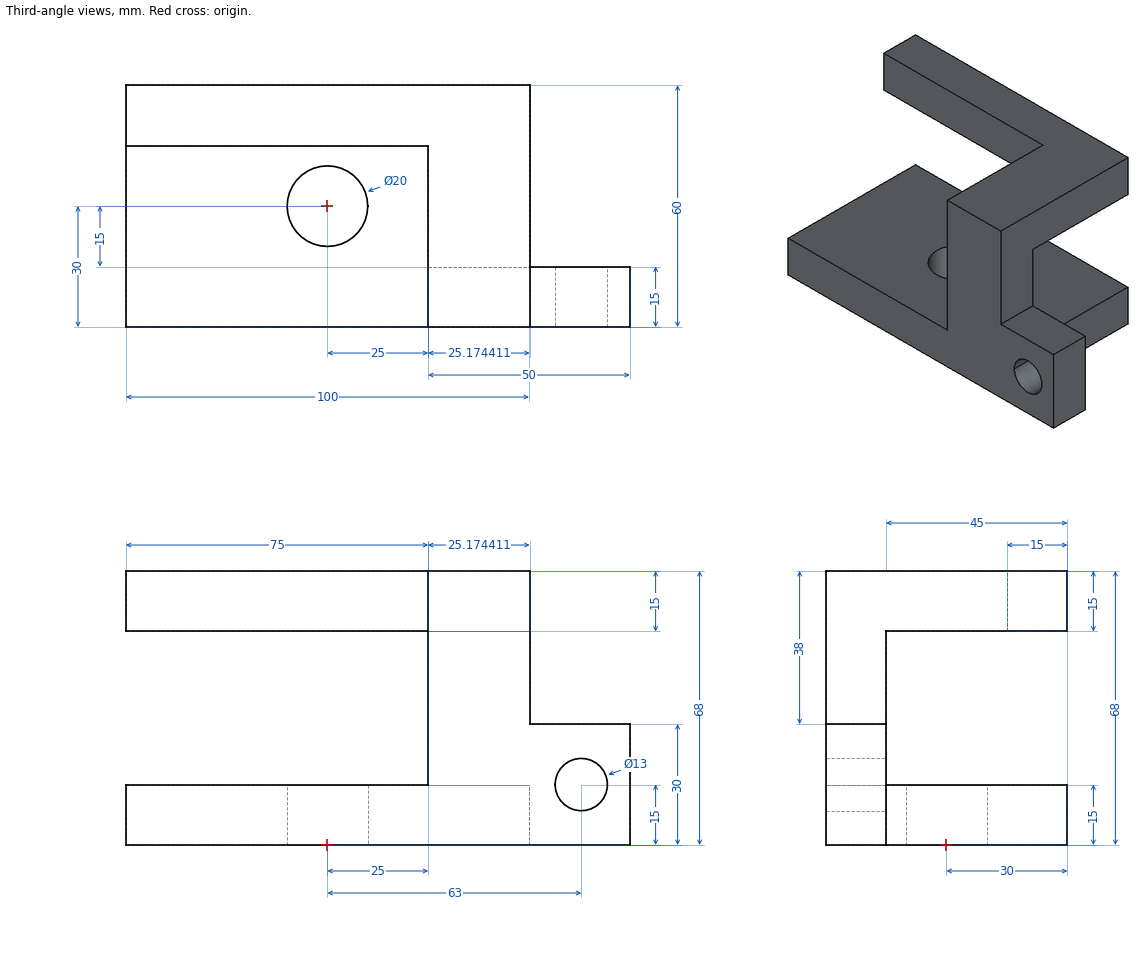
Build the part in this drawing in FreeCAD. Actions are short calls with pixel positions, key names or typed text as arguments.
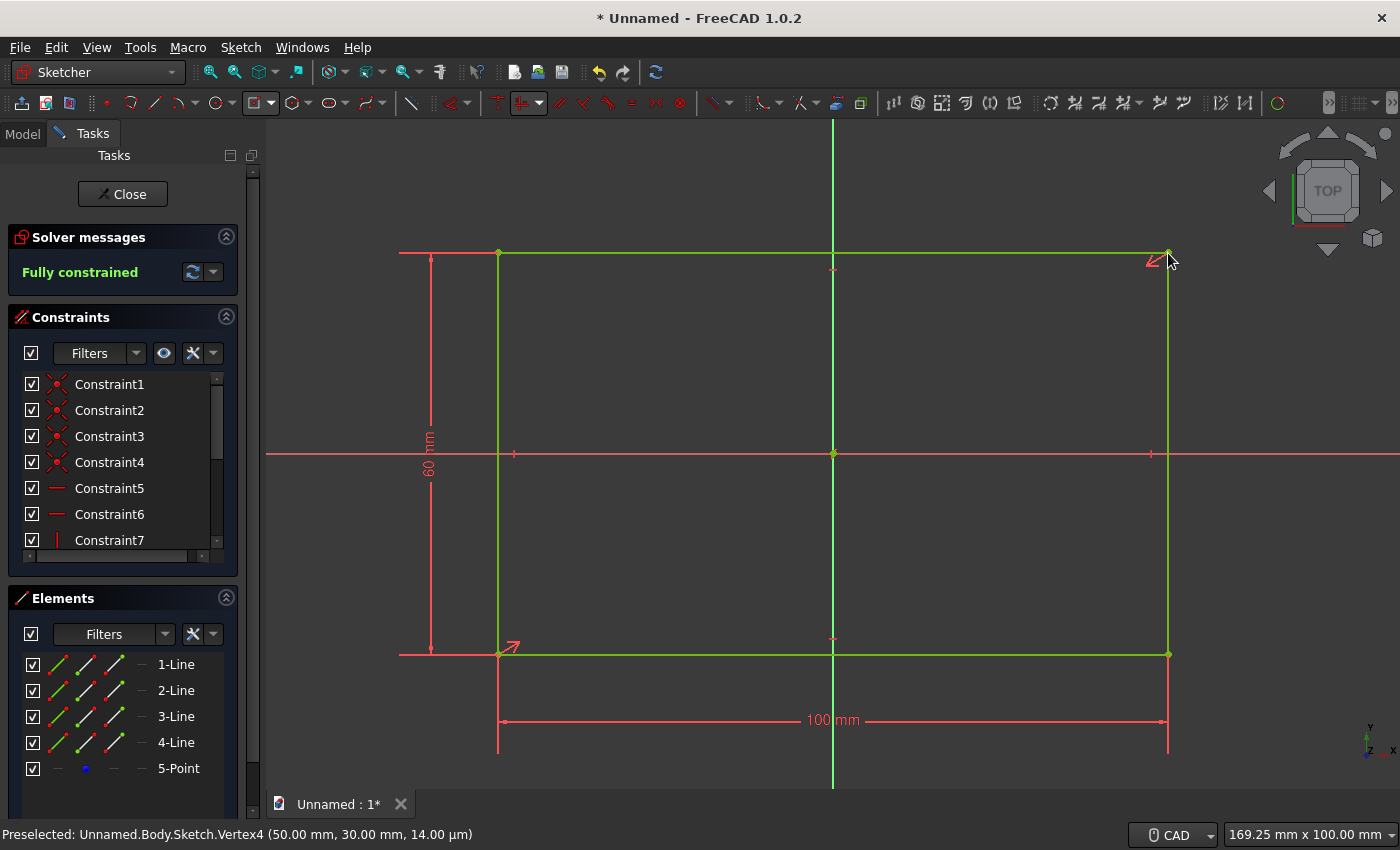
click(123, 194)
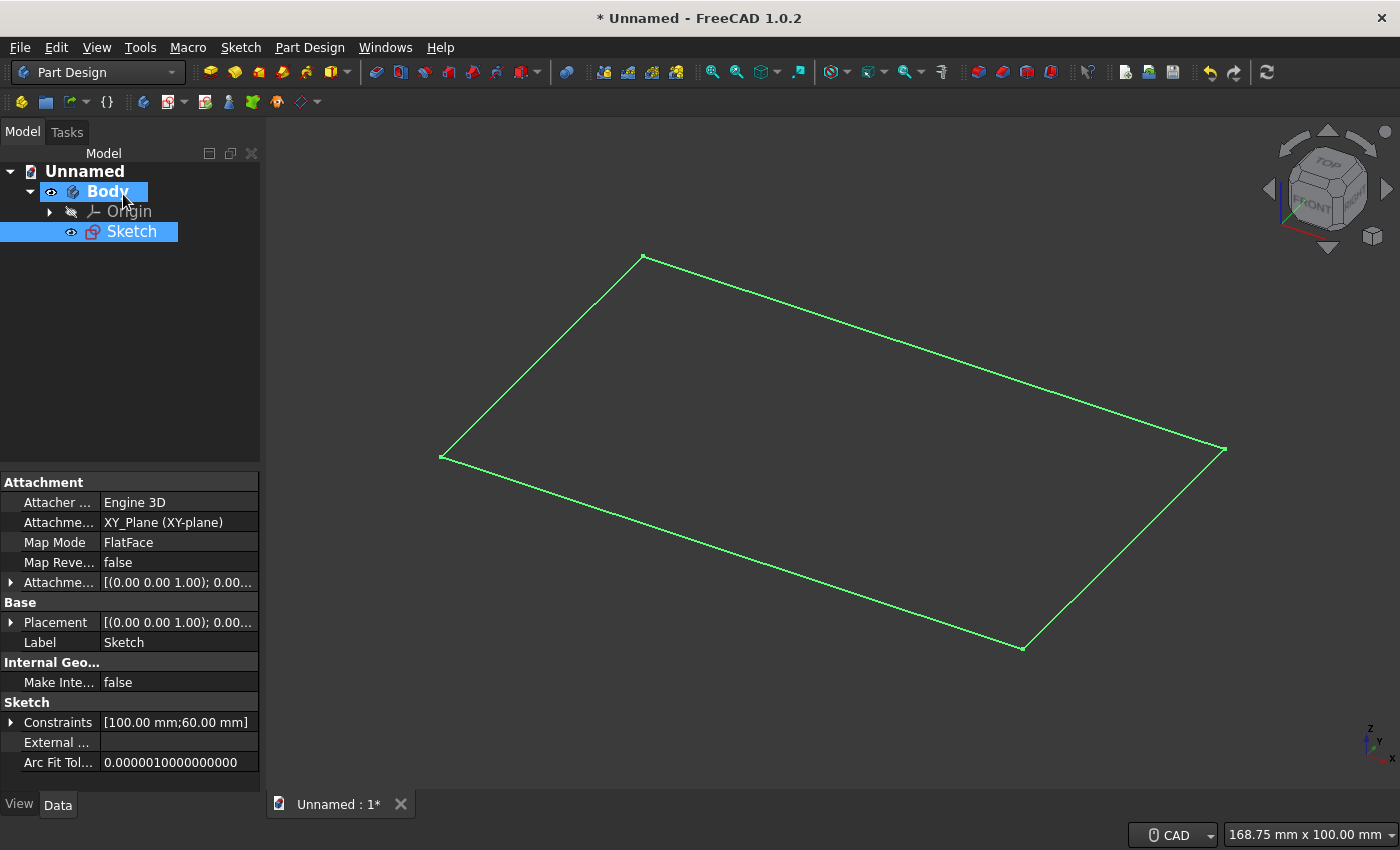
click(212, 72)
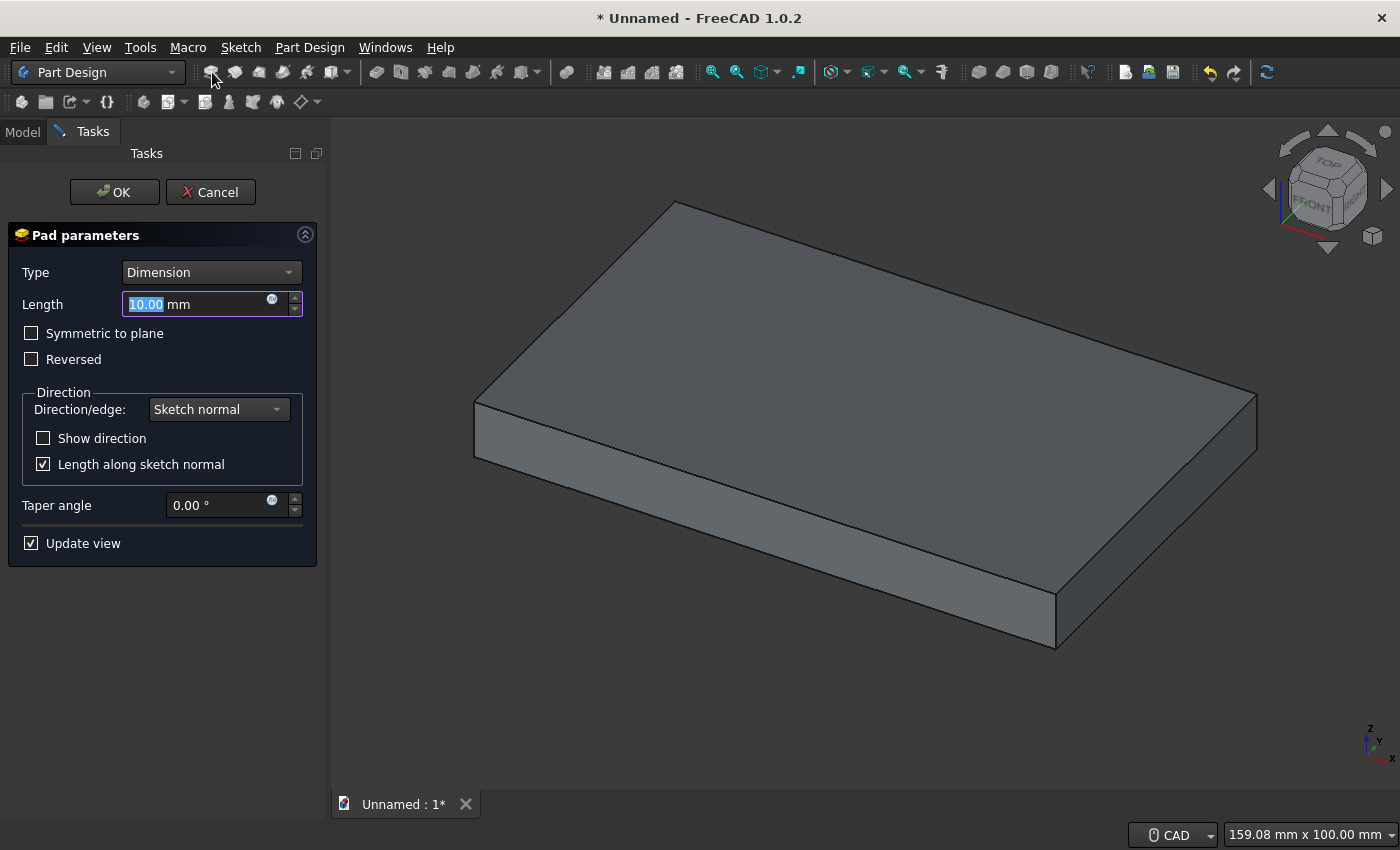
text(15)
key(Tab)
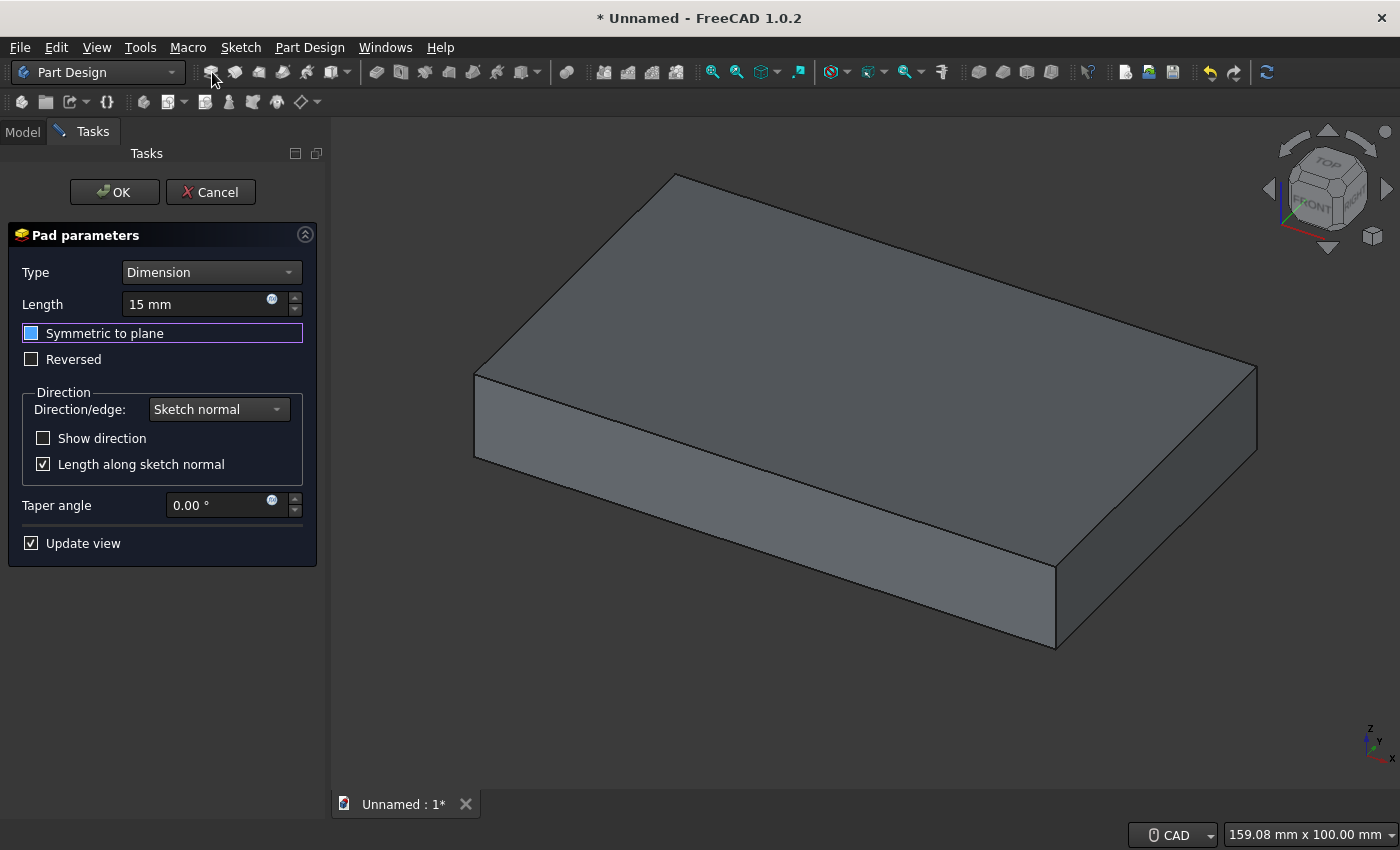
click(115, 192)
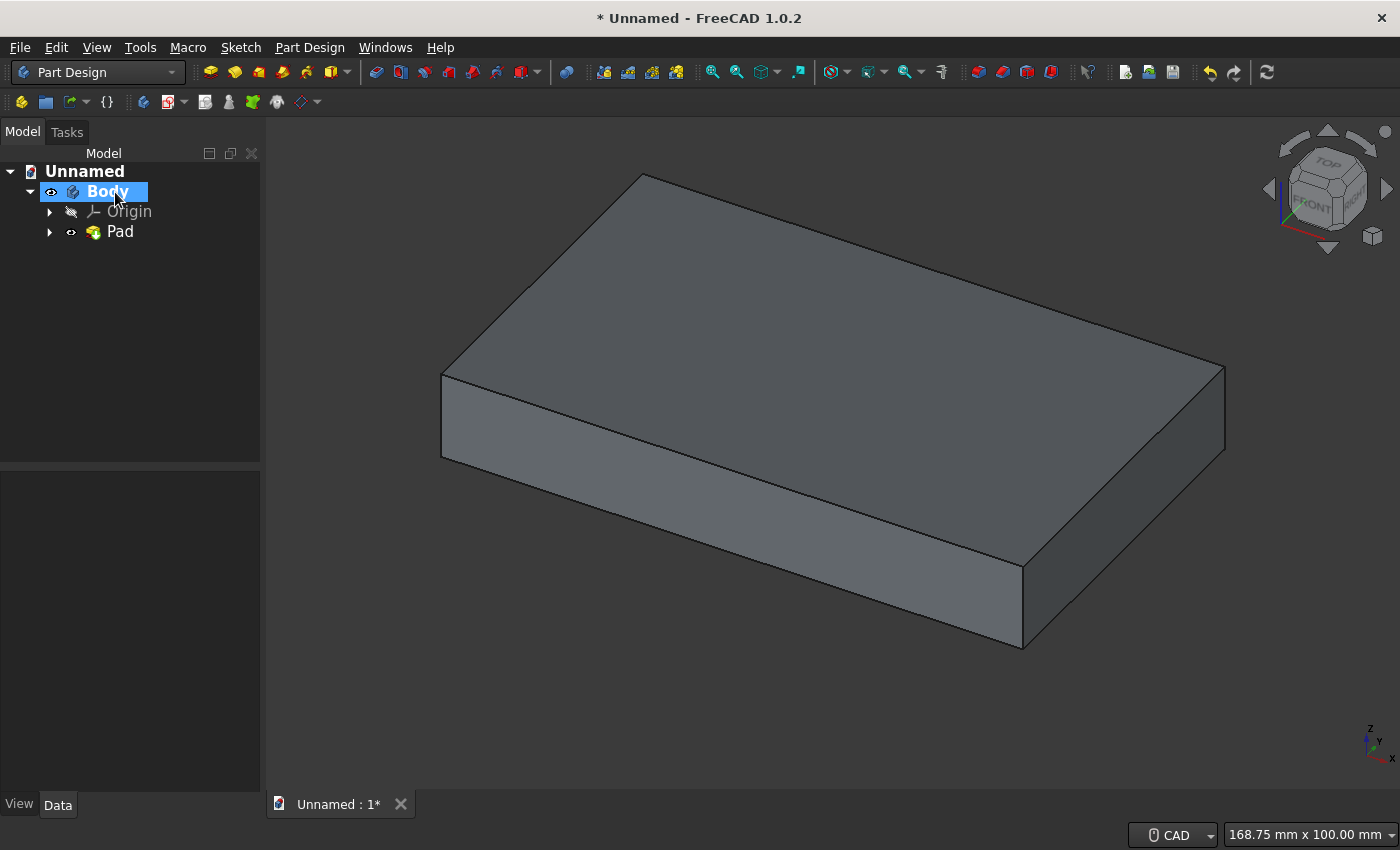
key(5)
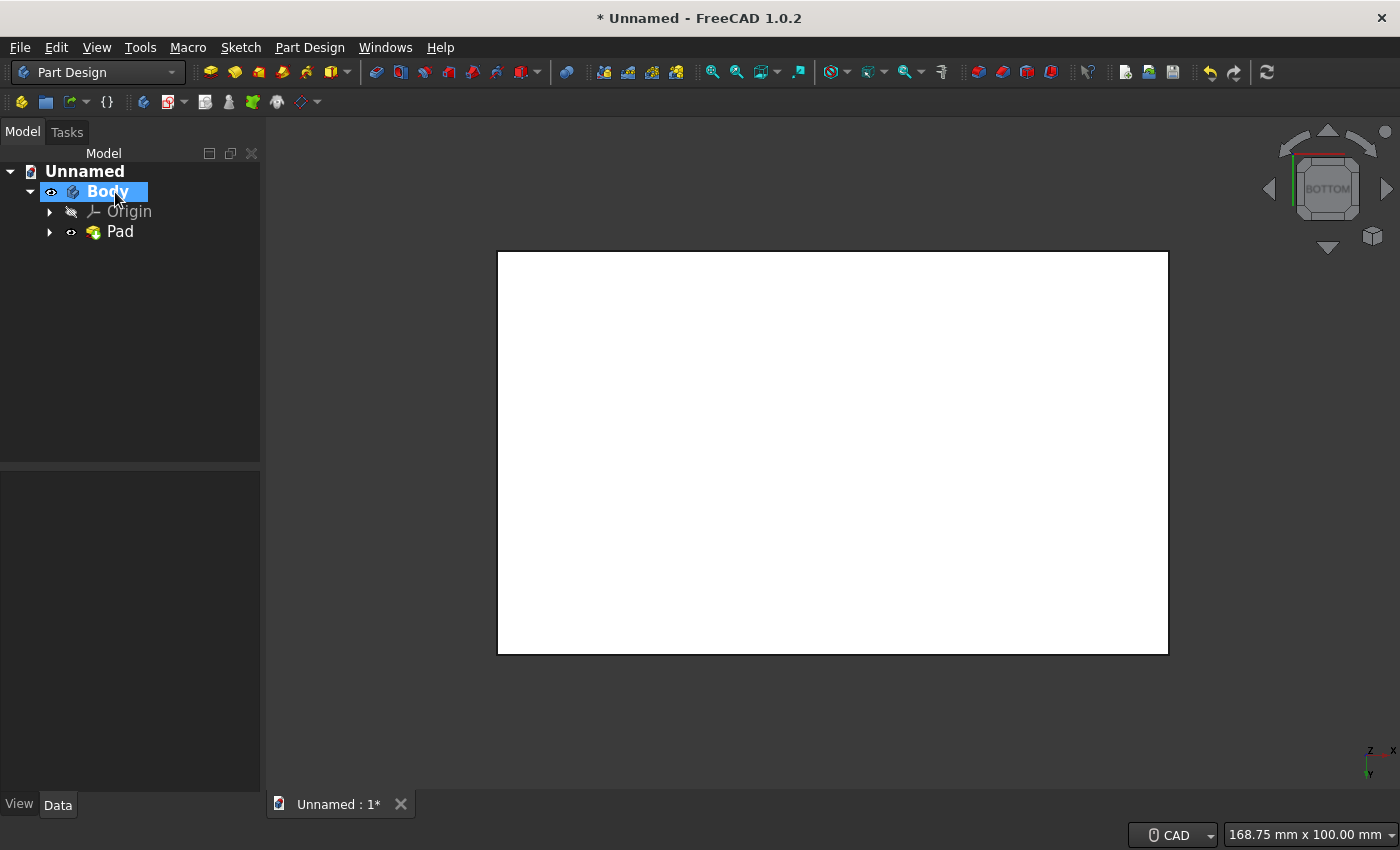
click(929, 452)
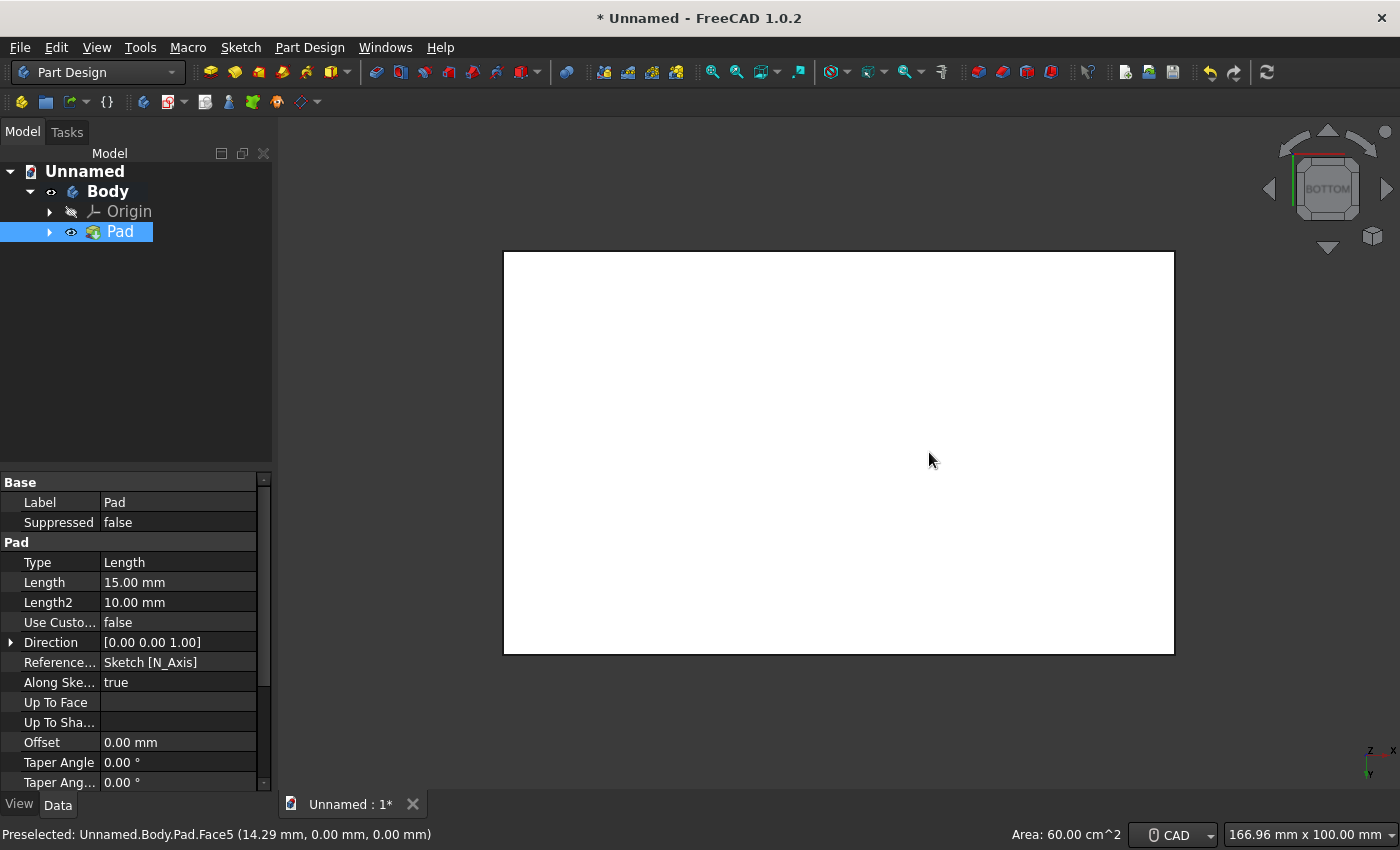
click(168, 102)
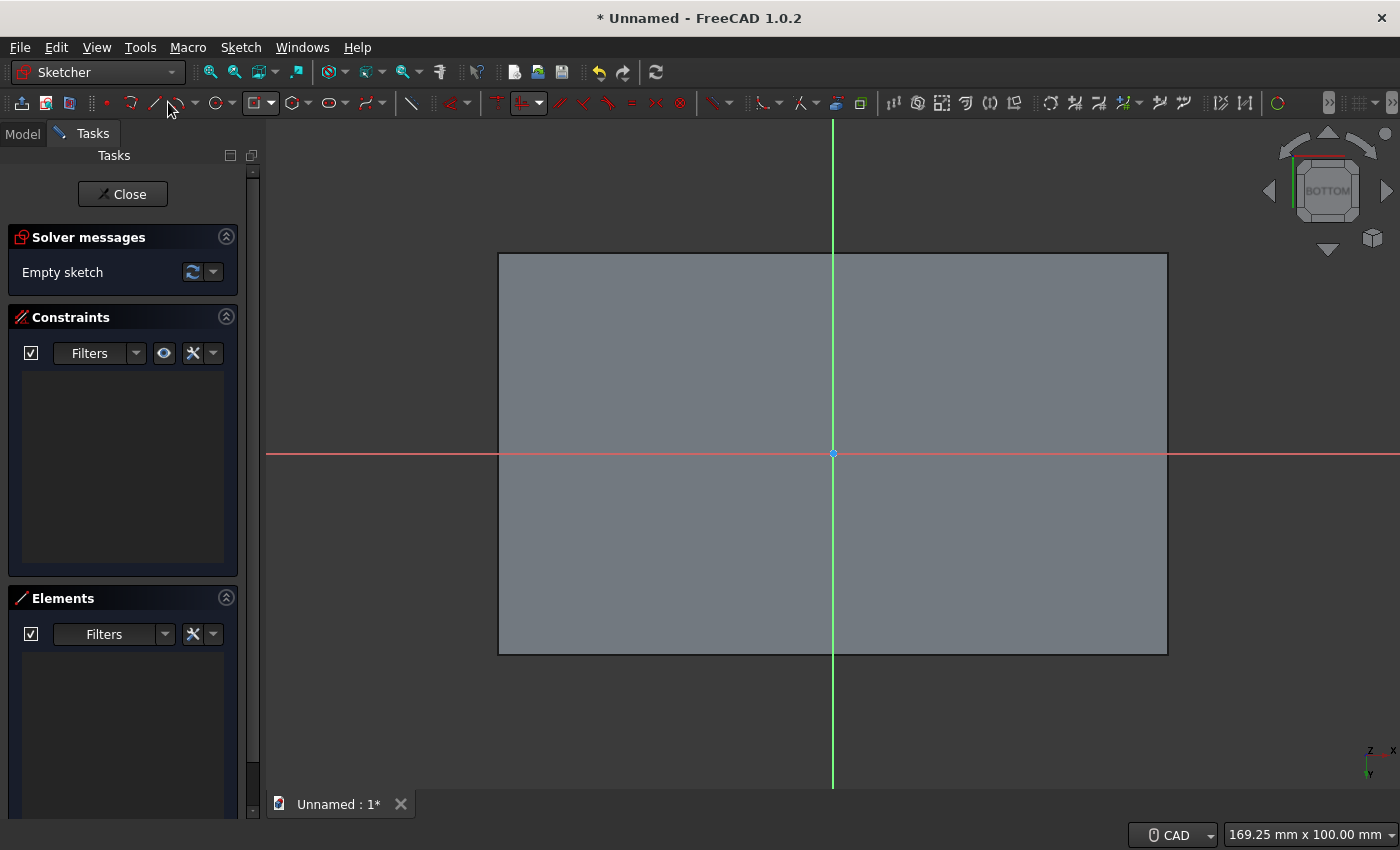
scroll(294, 761, down, 1)